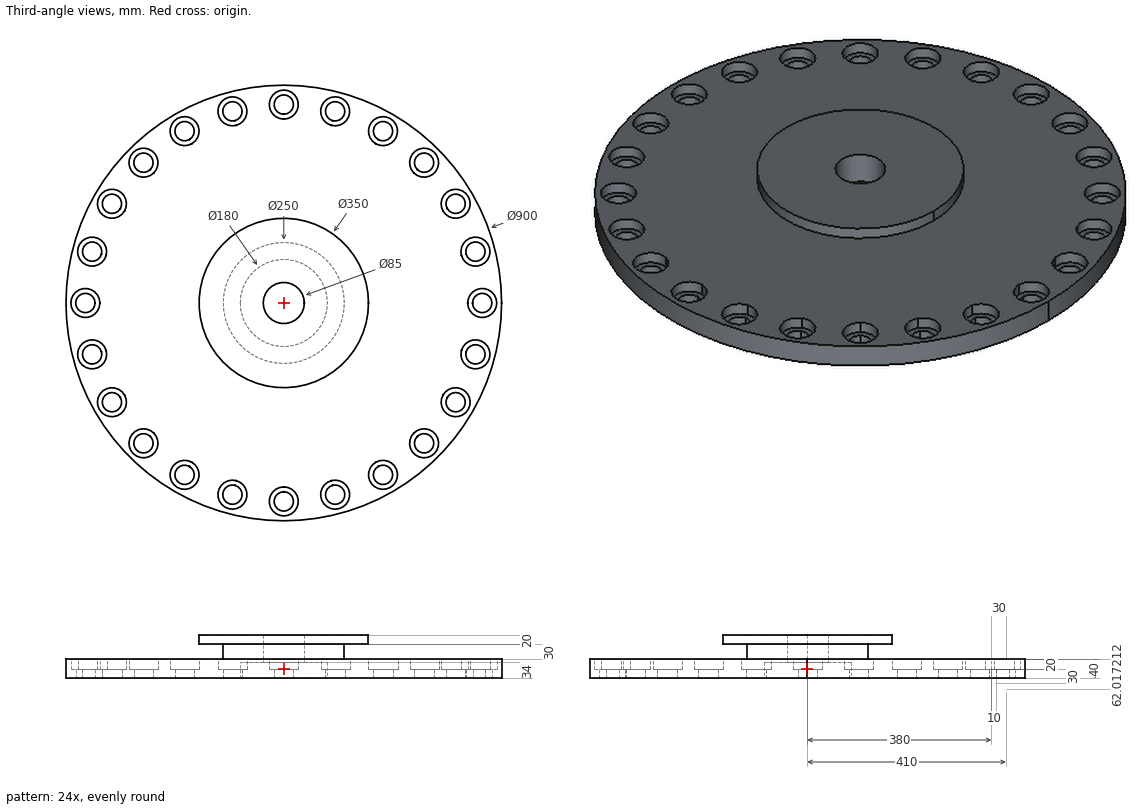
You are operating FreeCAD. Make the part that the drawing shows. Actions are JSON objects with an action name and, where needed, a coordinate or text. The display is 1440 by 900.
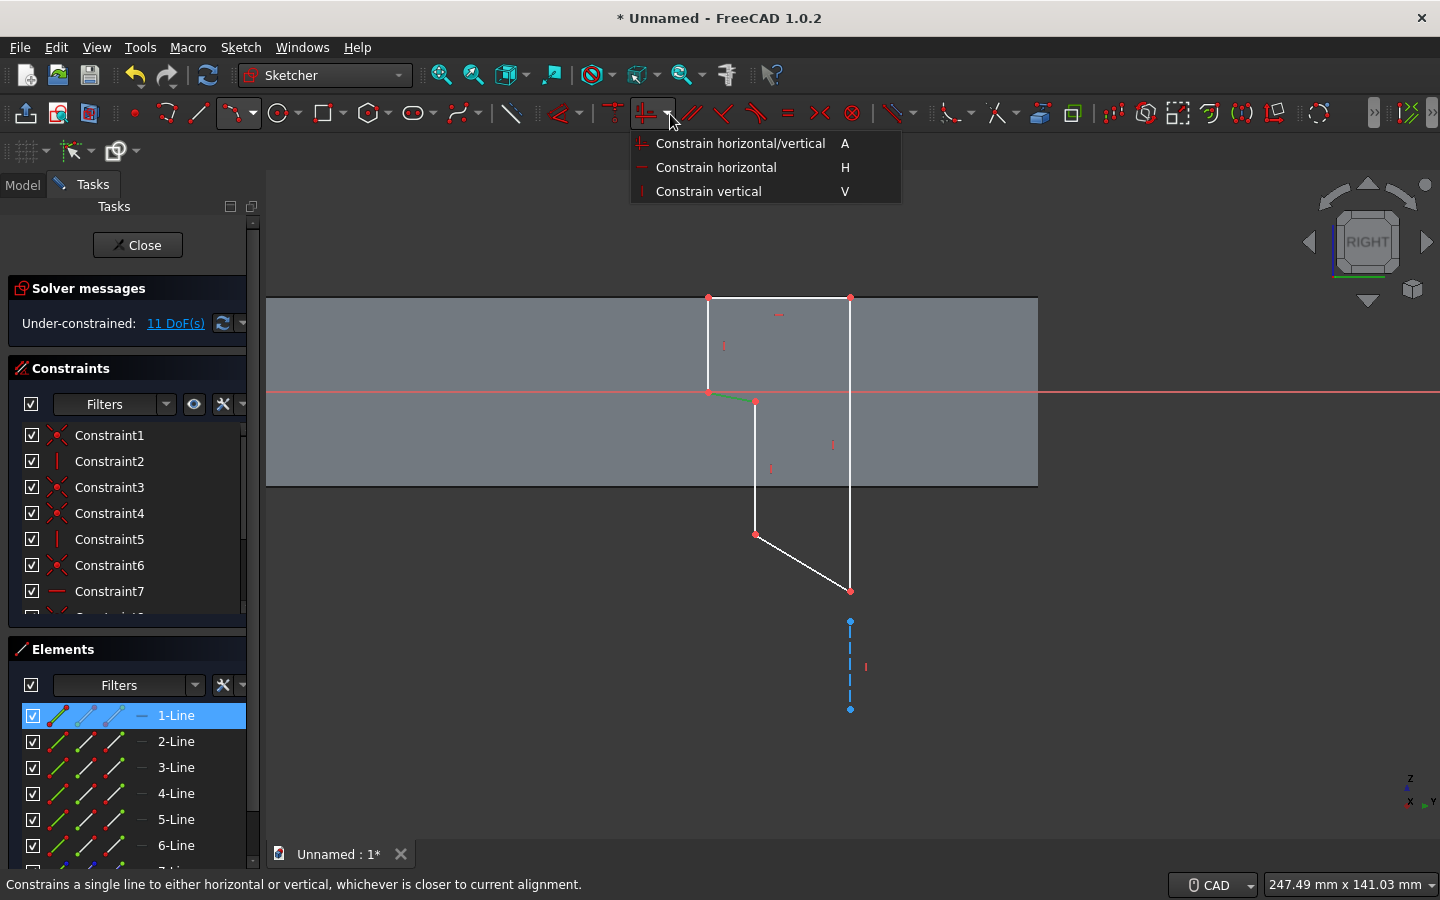
{"action": "left_click", "coordinate": [766, 167]}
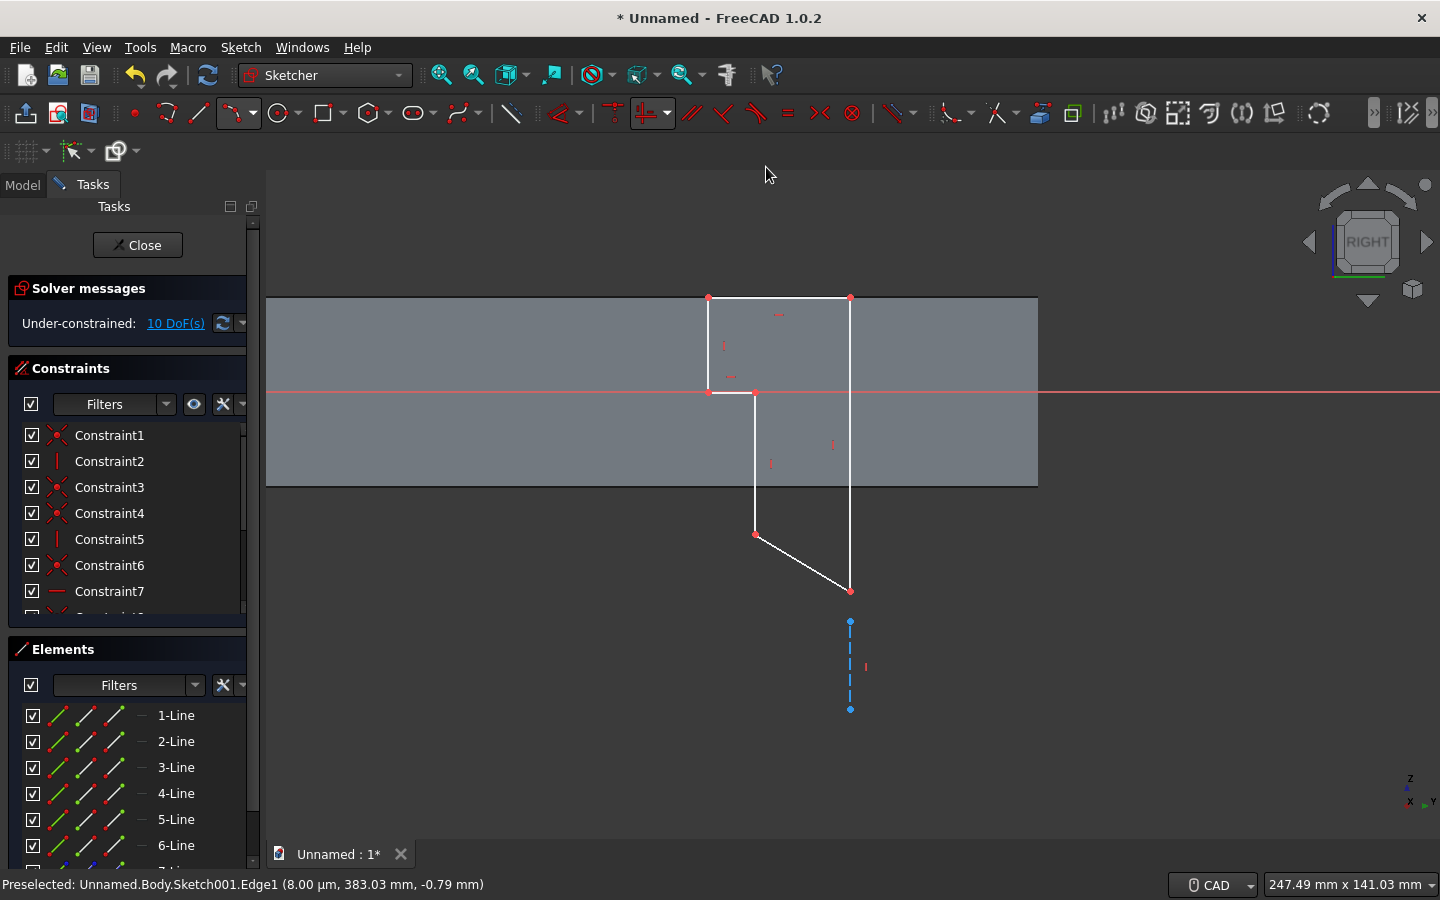
{"action": "left_click", "coordinate": [708, 393]}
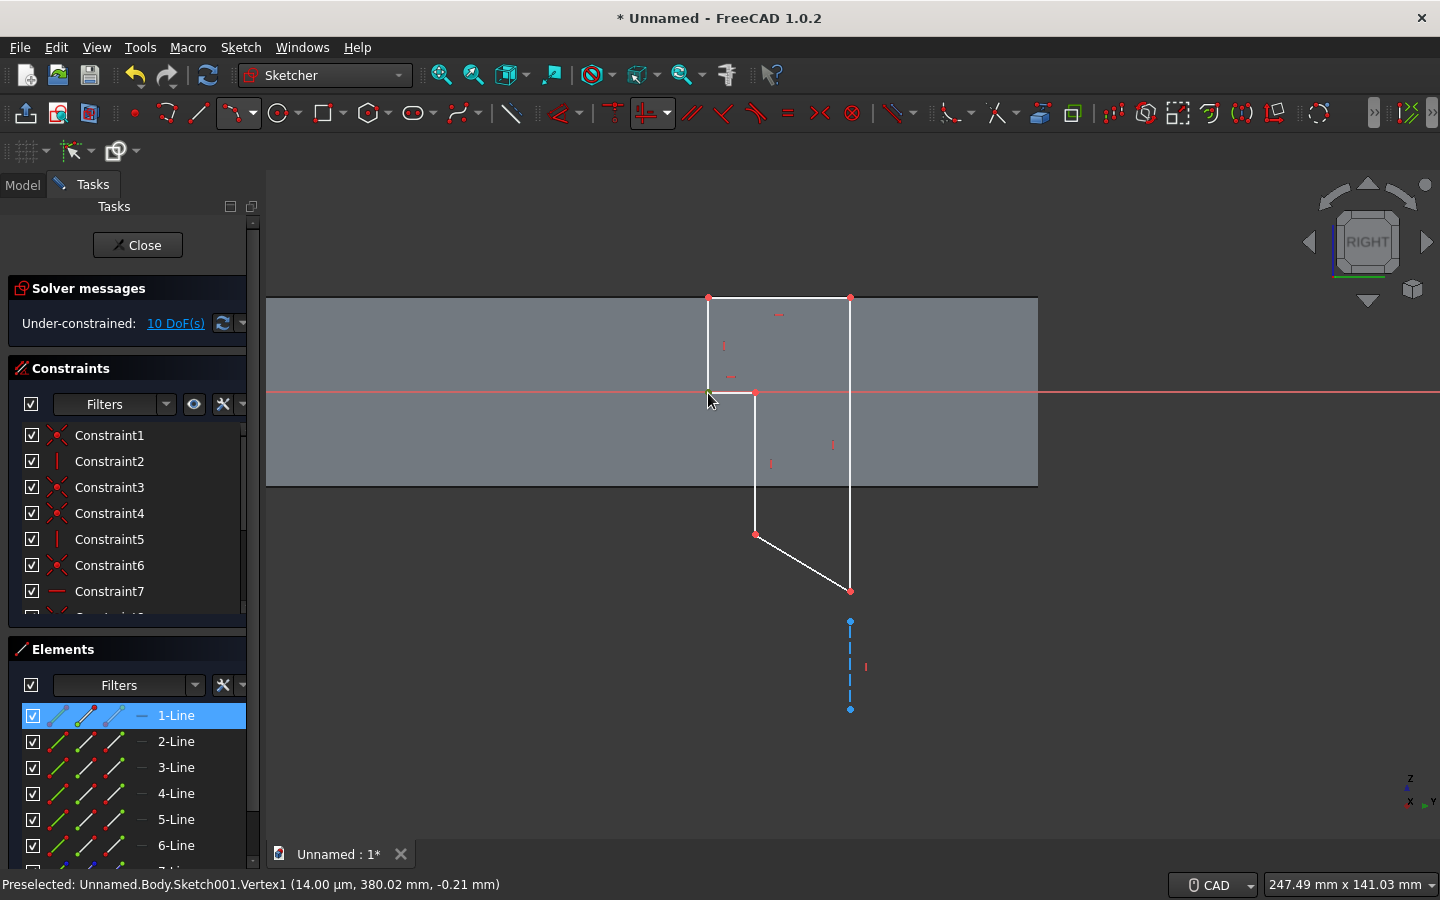
{"action": "left_click", "coordinate": [364, 392]}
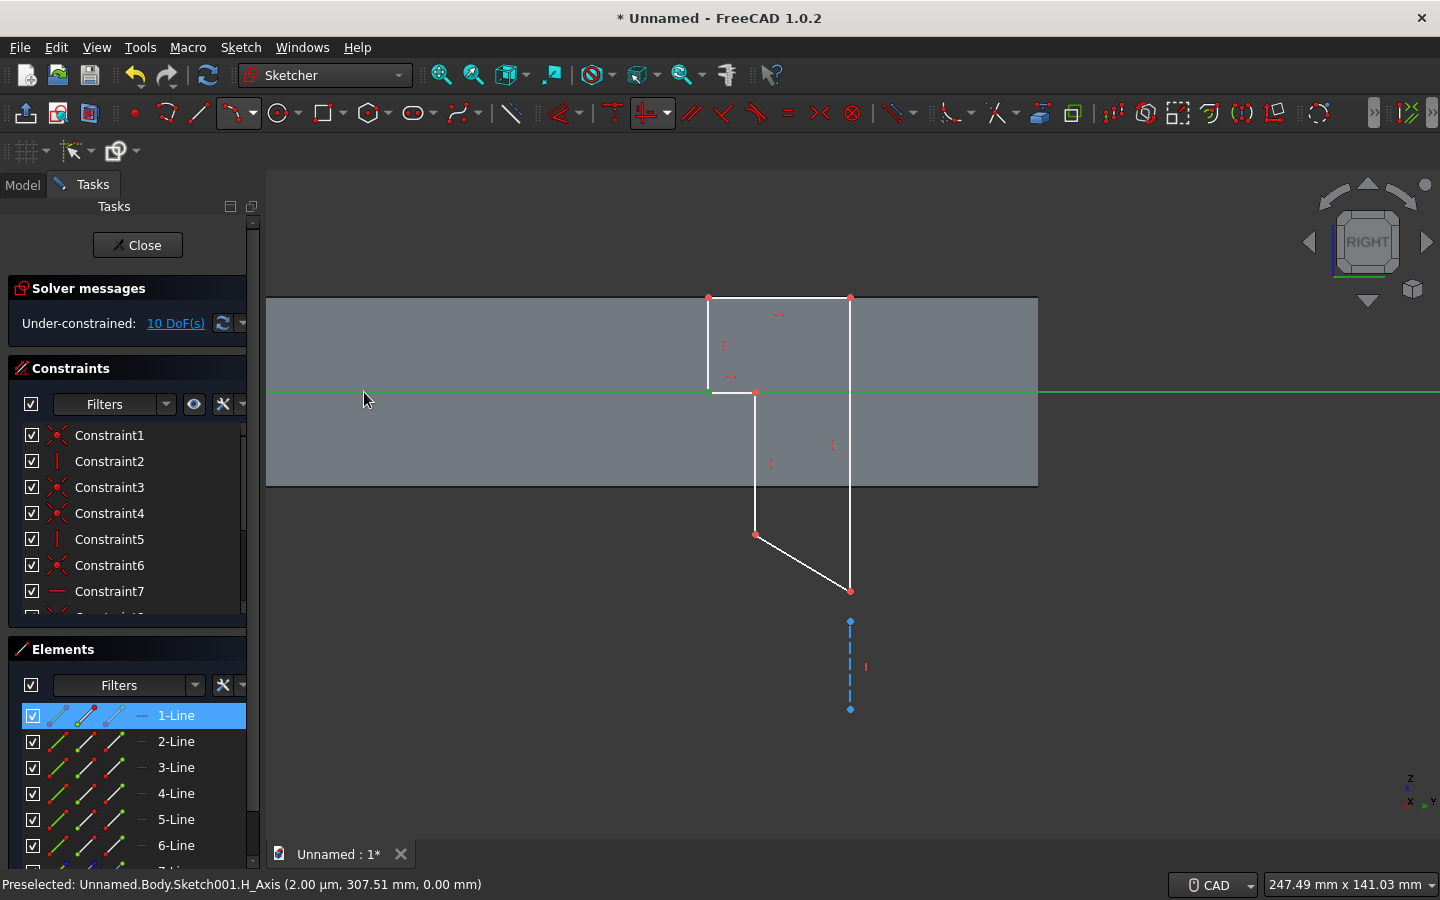
{"action": "left_click", "coordinate": [614, 114]}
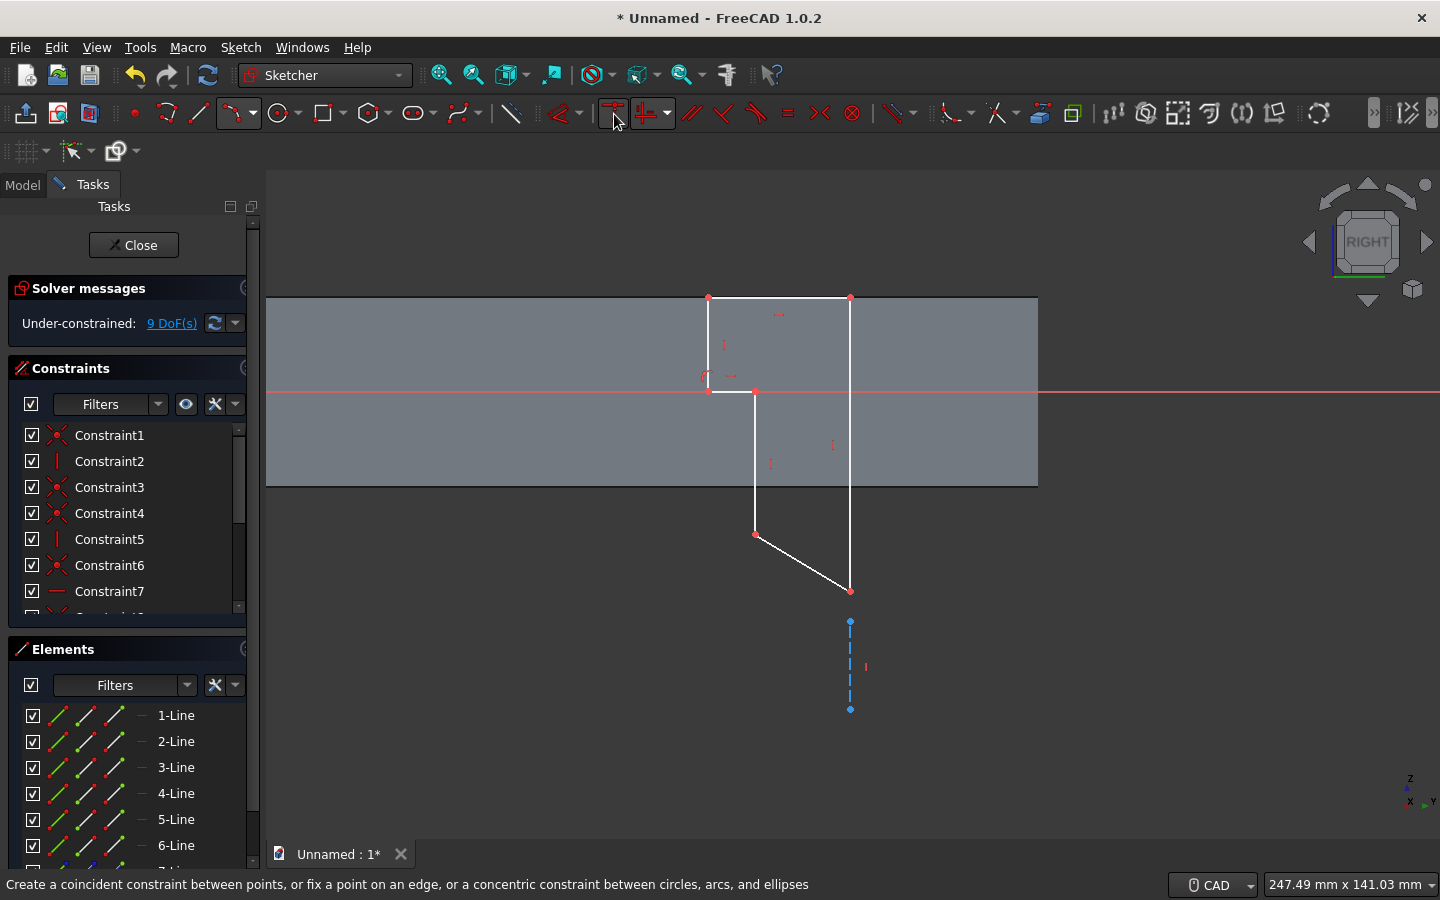
{"action": "left_click", "coordinate": [722, 392]}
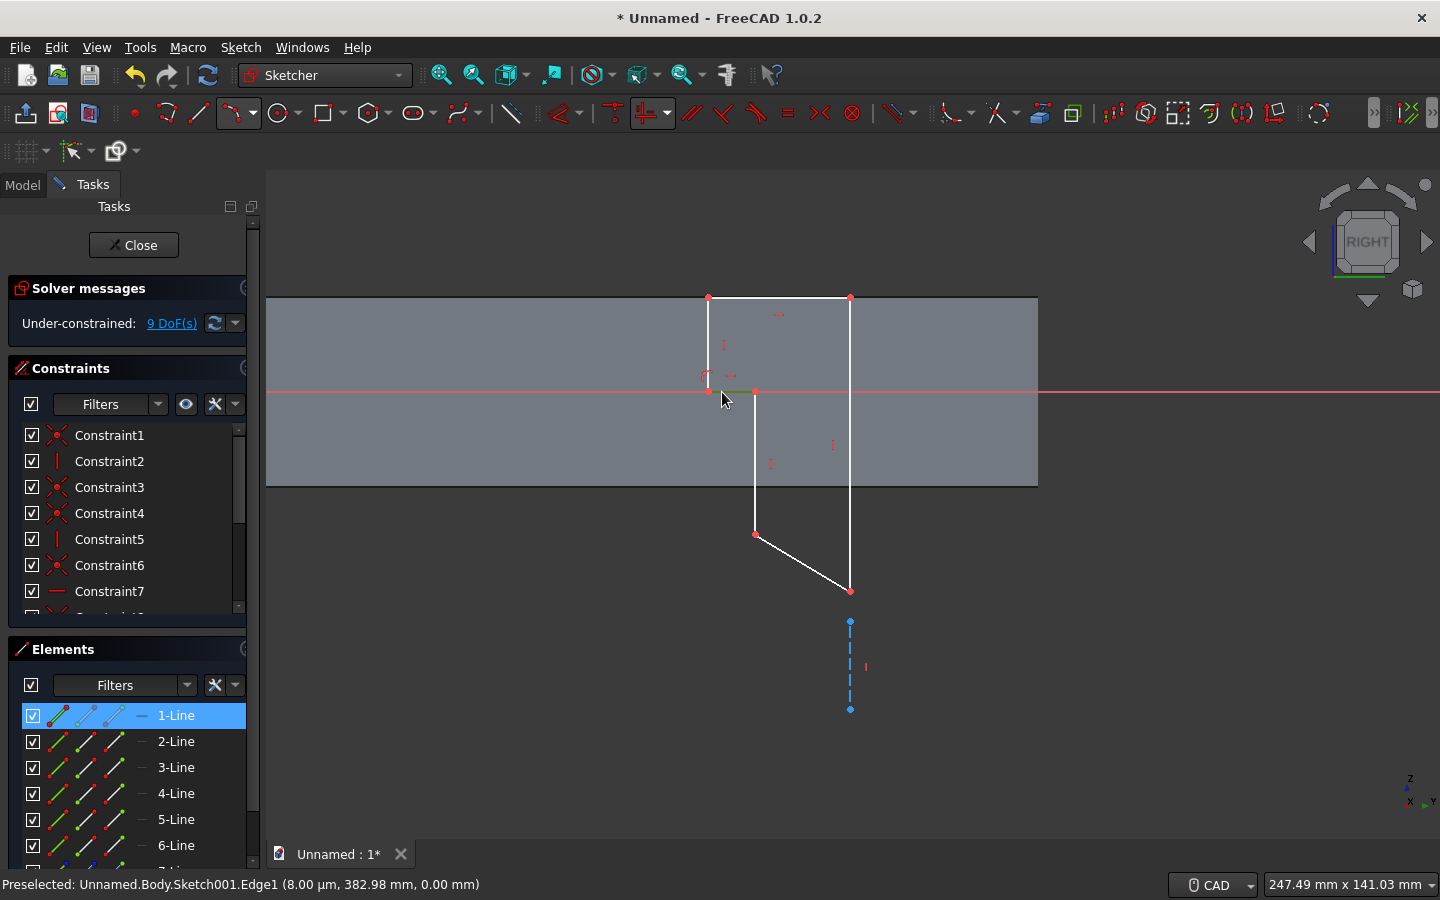
{"action": "key", "text": "l"}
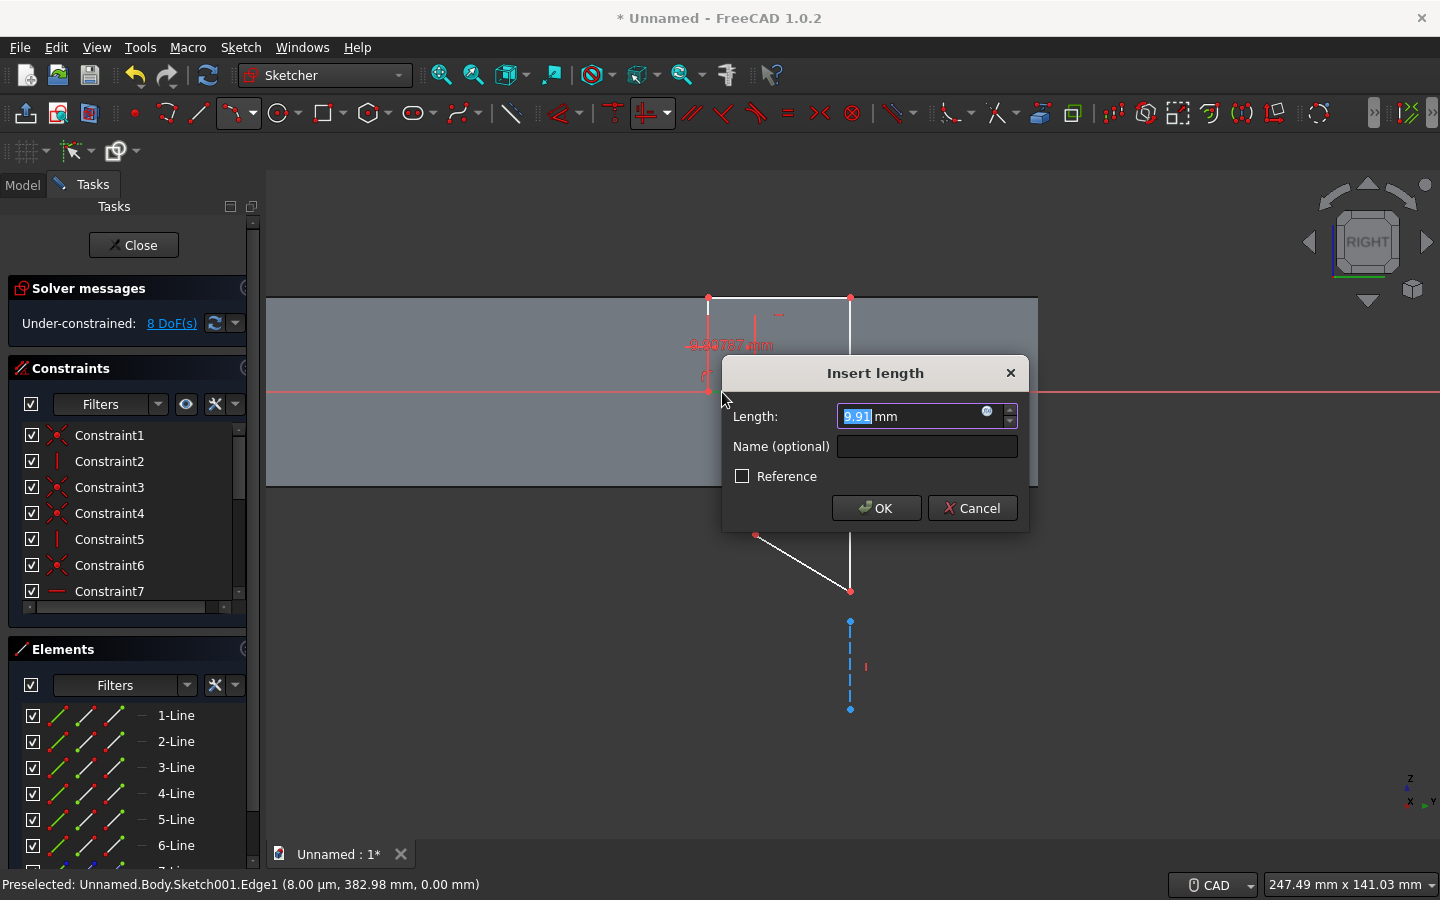
{"action": "type", "text": "10"}
{"action": "key", "text": "Return"}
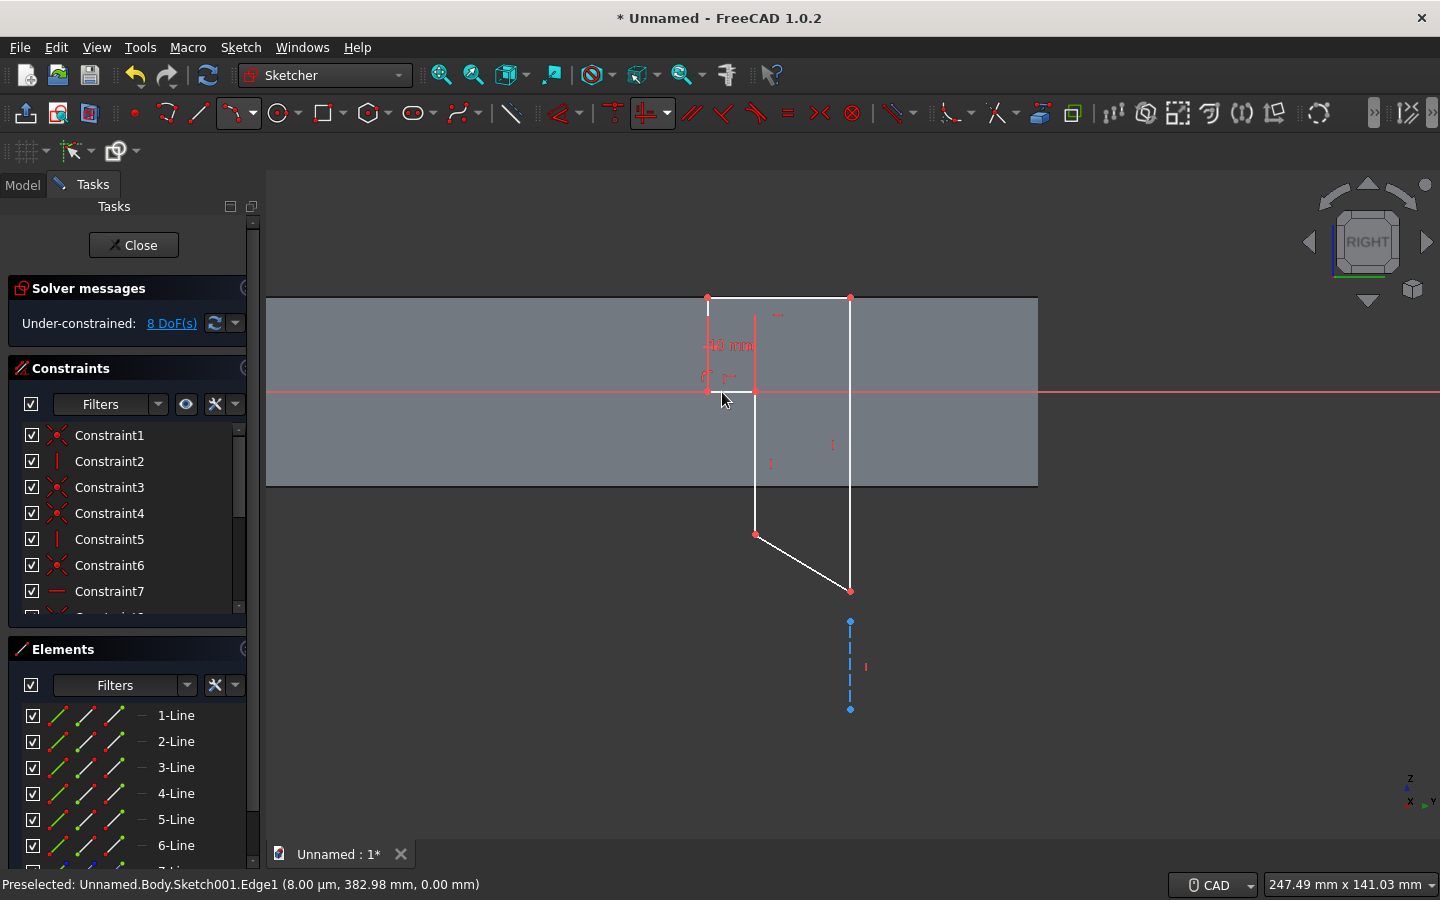
{"action": "left_click", "coordinate": [755, 435]}